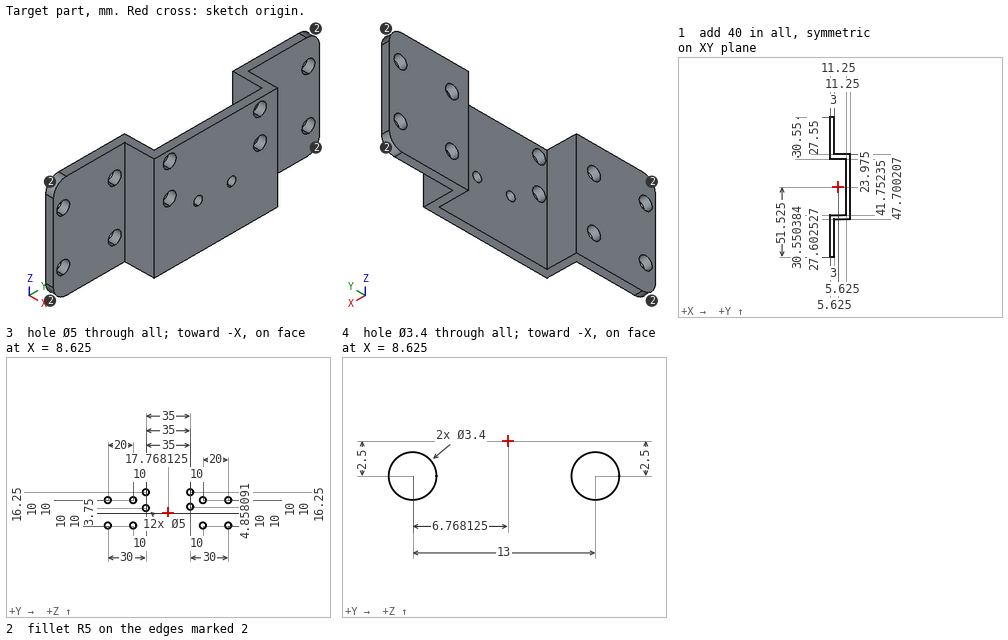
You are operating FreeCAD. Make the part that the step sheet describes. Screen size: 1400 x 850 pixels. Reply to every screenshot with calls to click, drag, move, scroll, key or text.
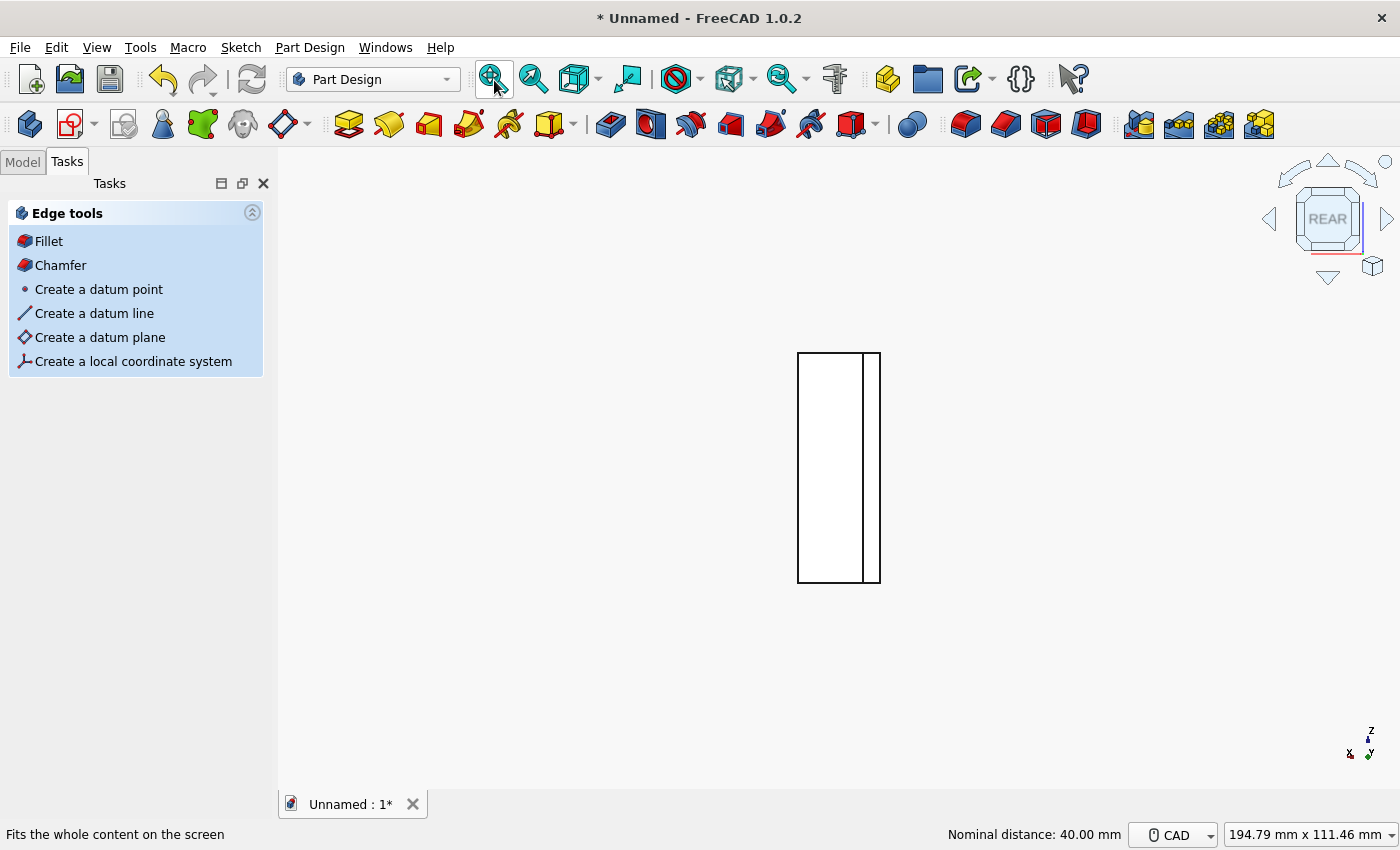
click(494, 80)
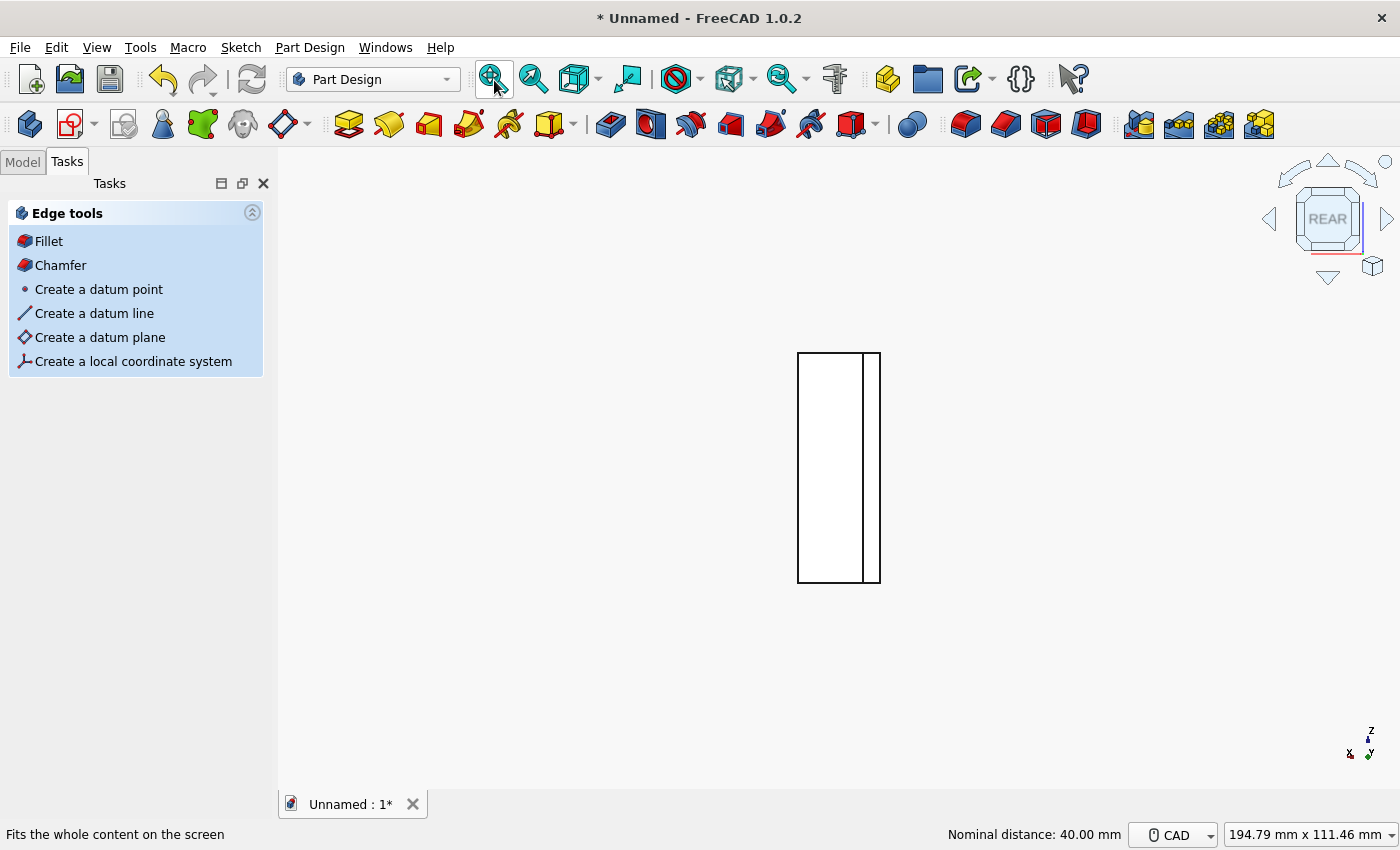
click(871, 582, ctrl)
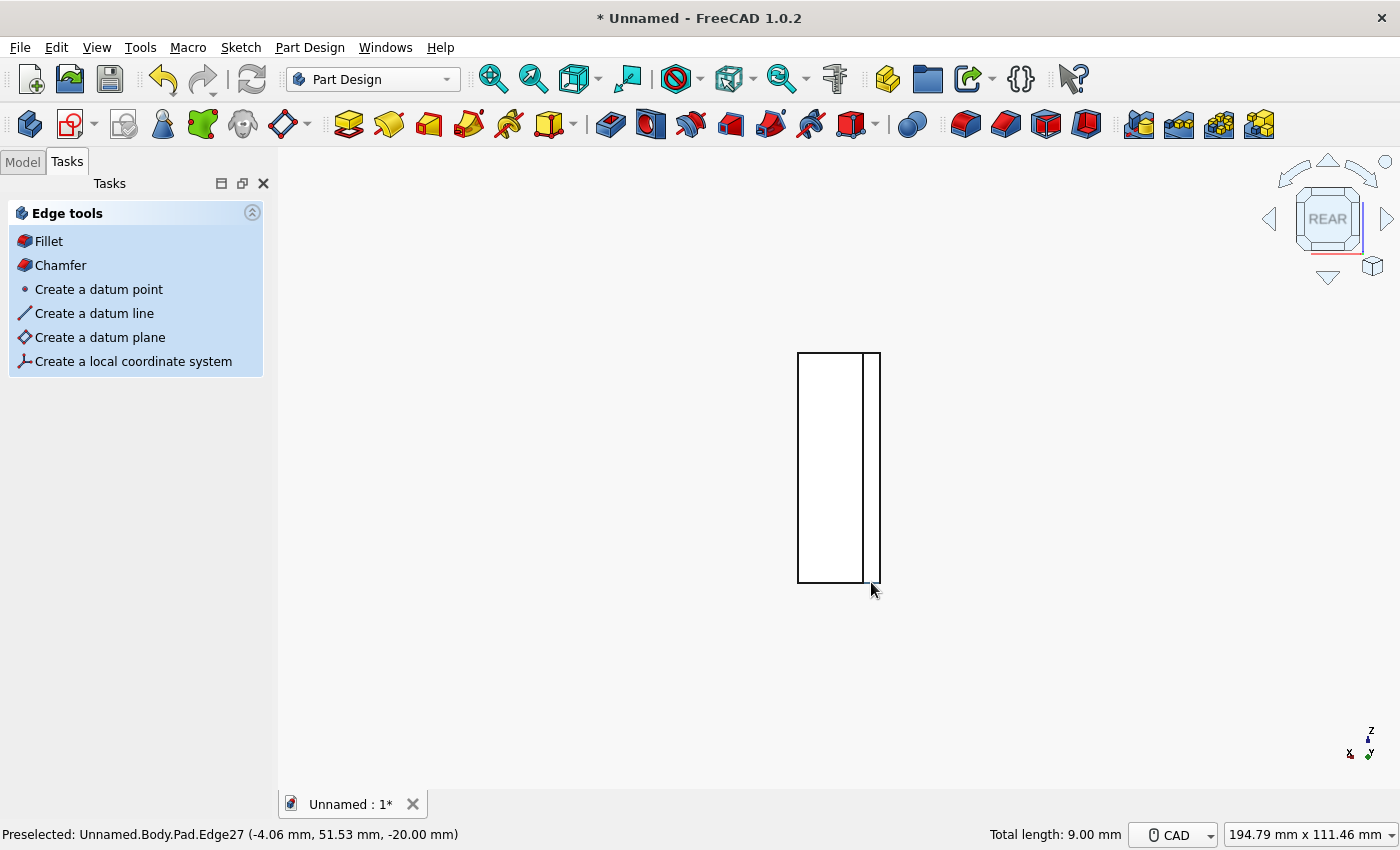
click(871, 352, ctrl)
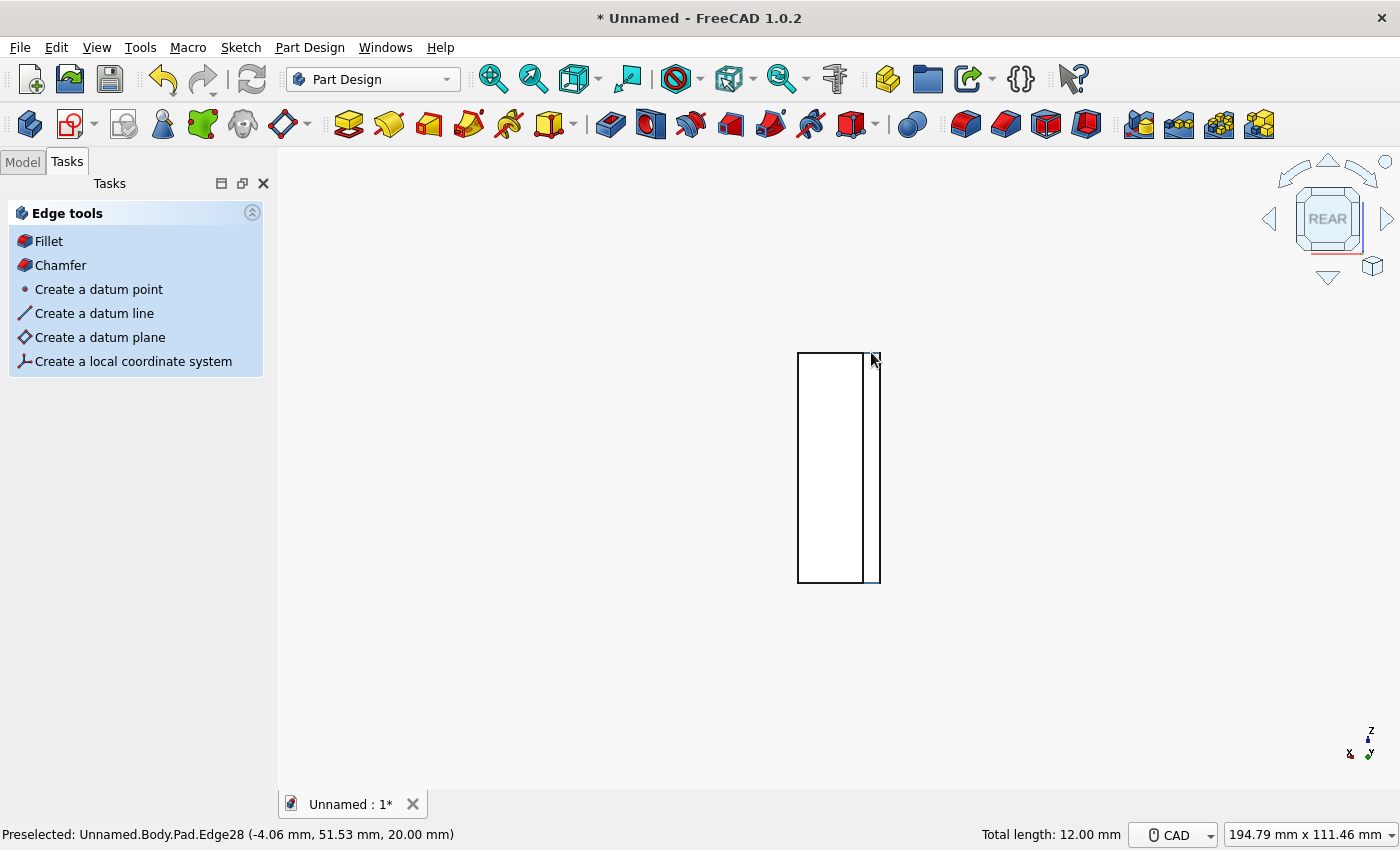
click(966, 124)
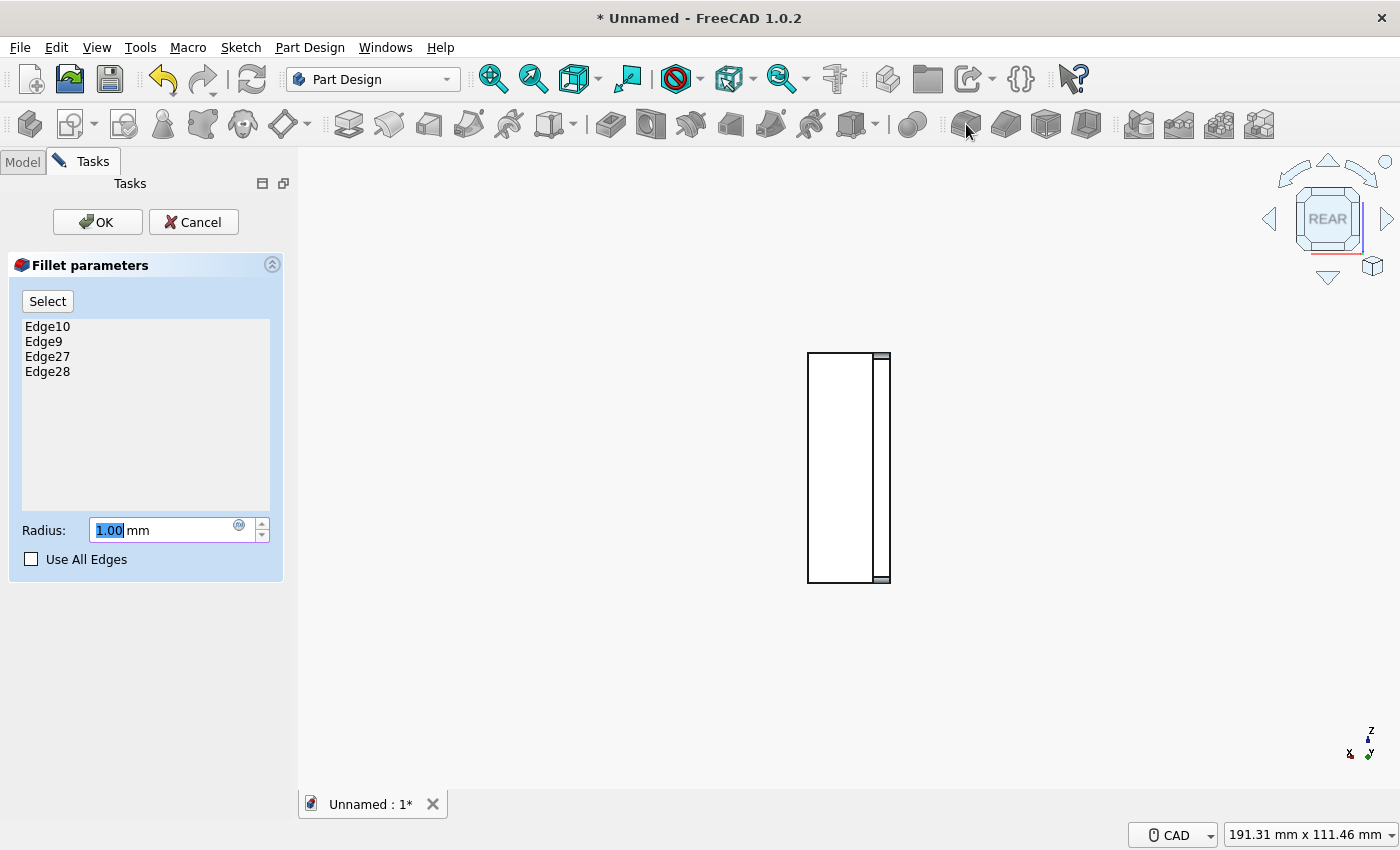
text(5)
key(Tab)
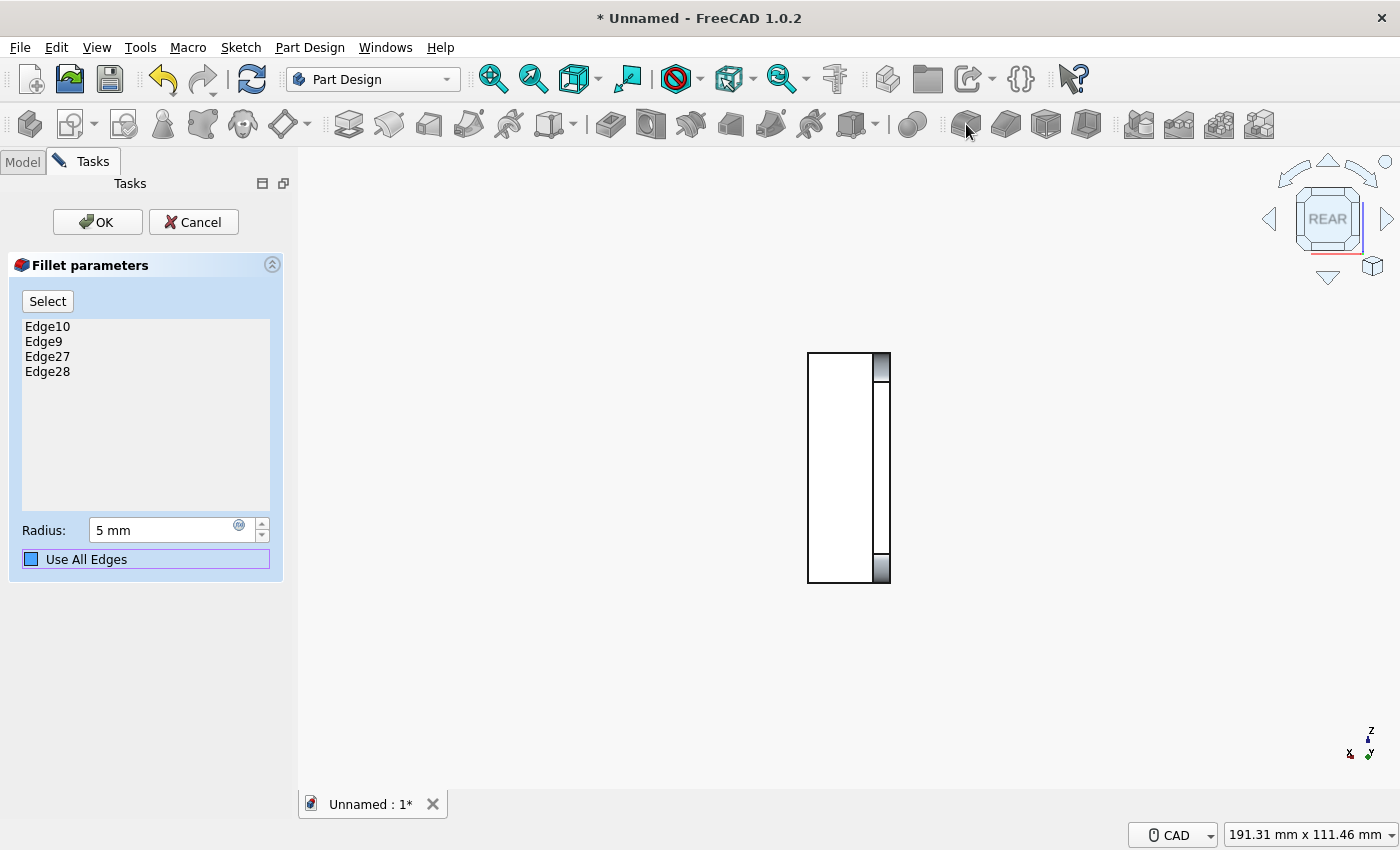
click(98, 222)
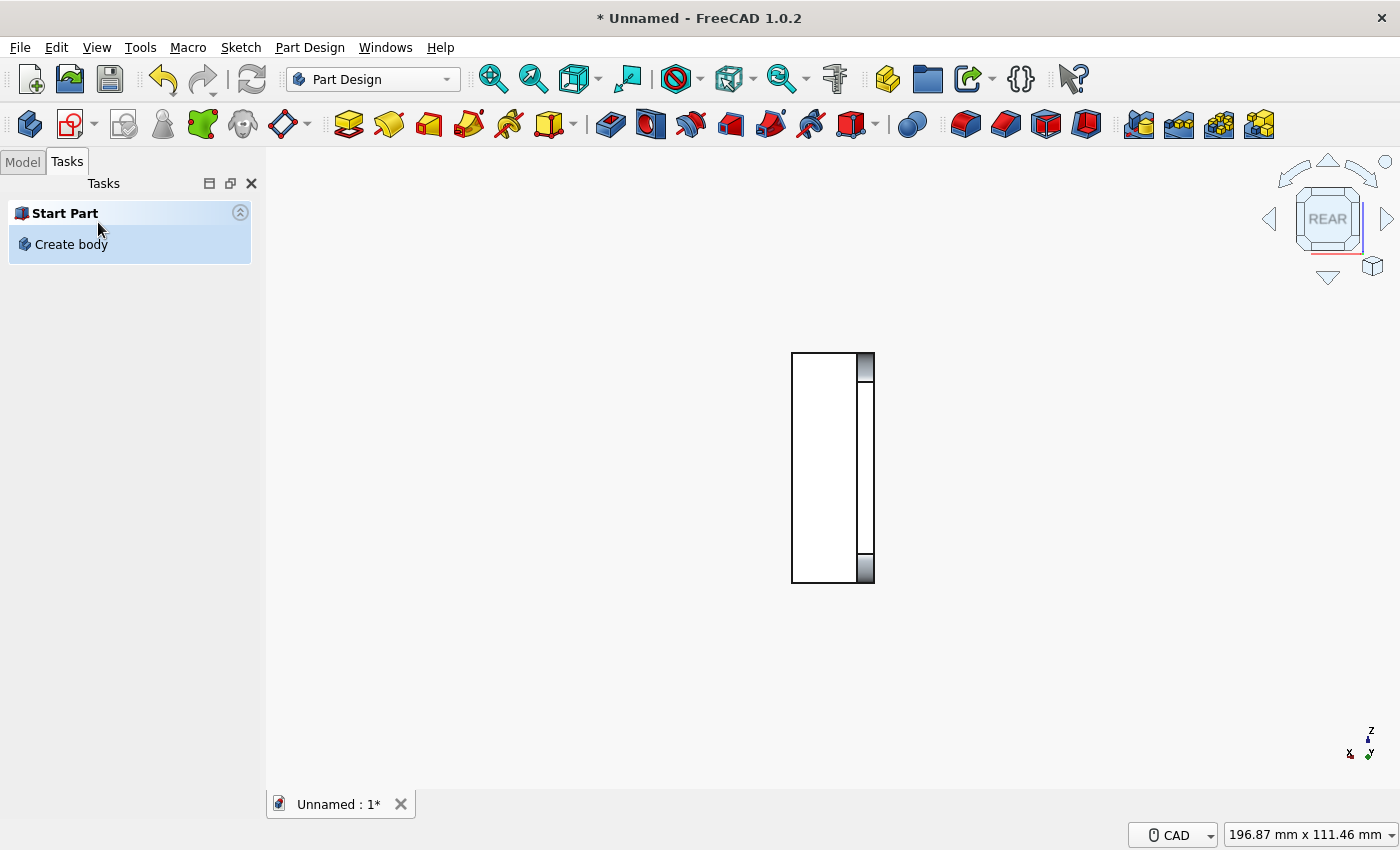
click(494, 80)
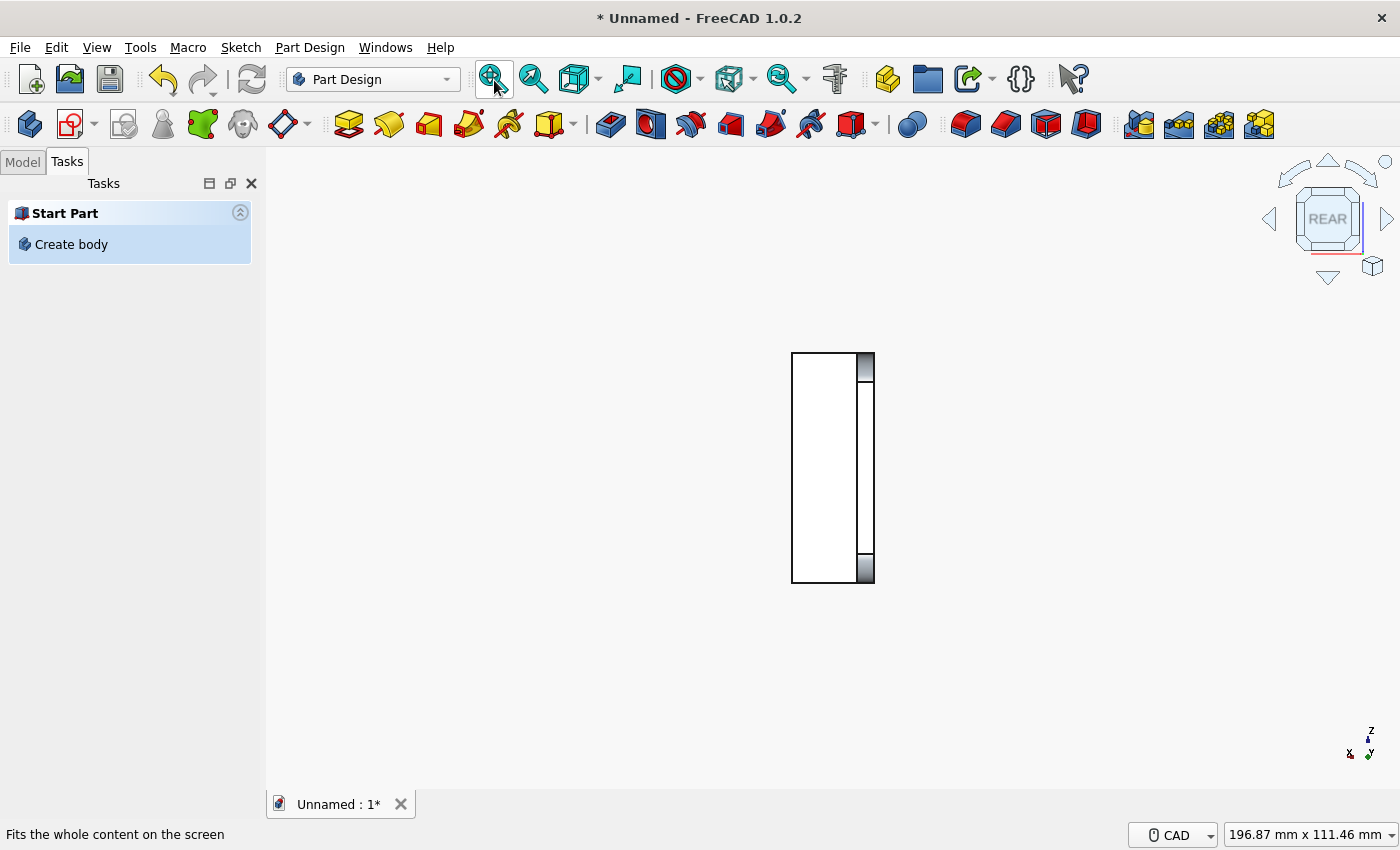
key(0)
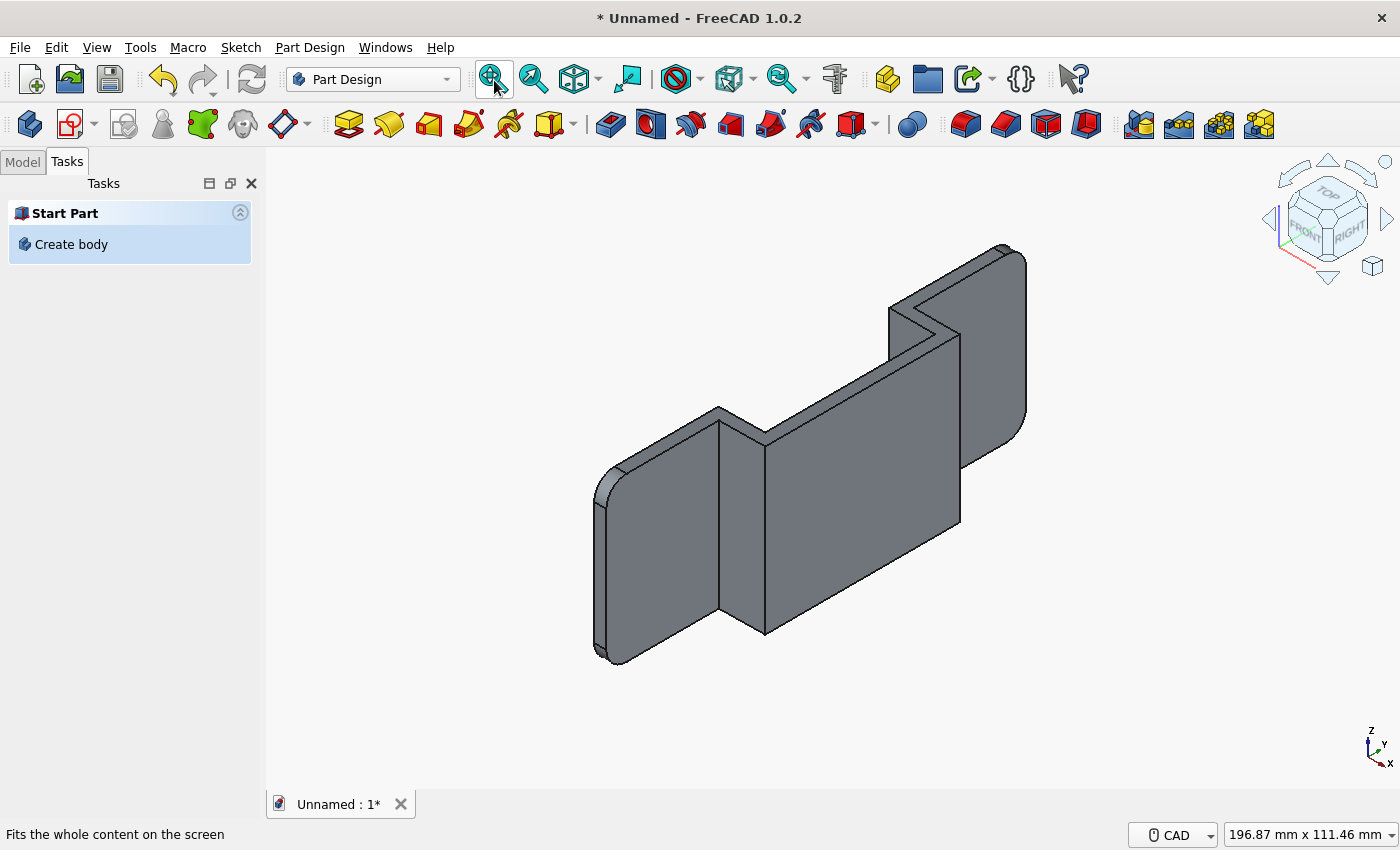
click(863, 483)